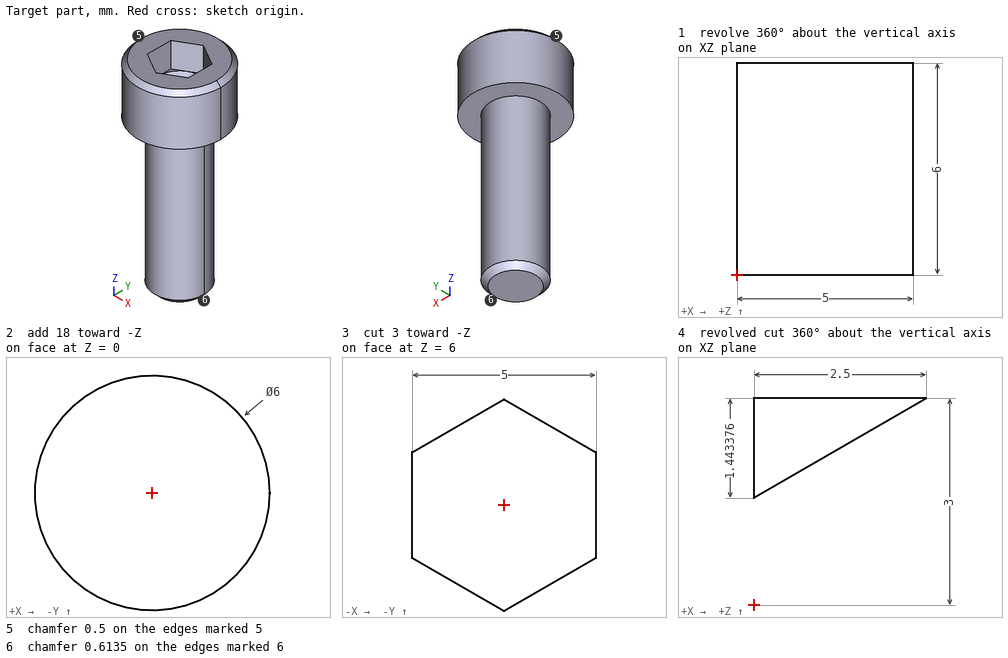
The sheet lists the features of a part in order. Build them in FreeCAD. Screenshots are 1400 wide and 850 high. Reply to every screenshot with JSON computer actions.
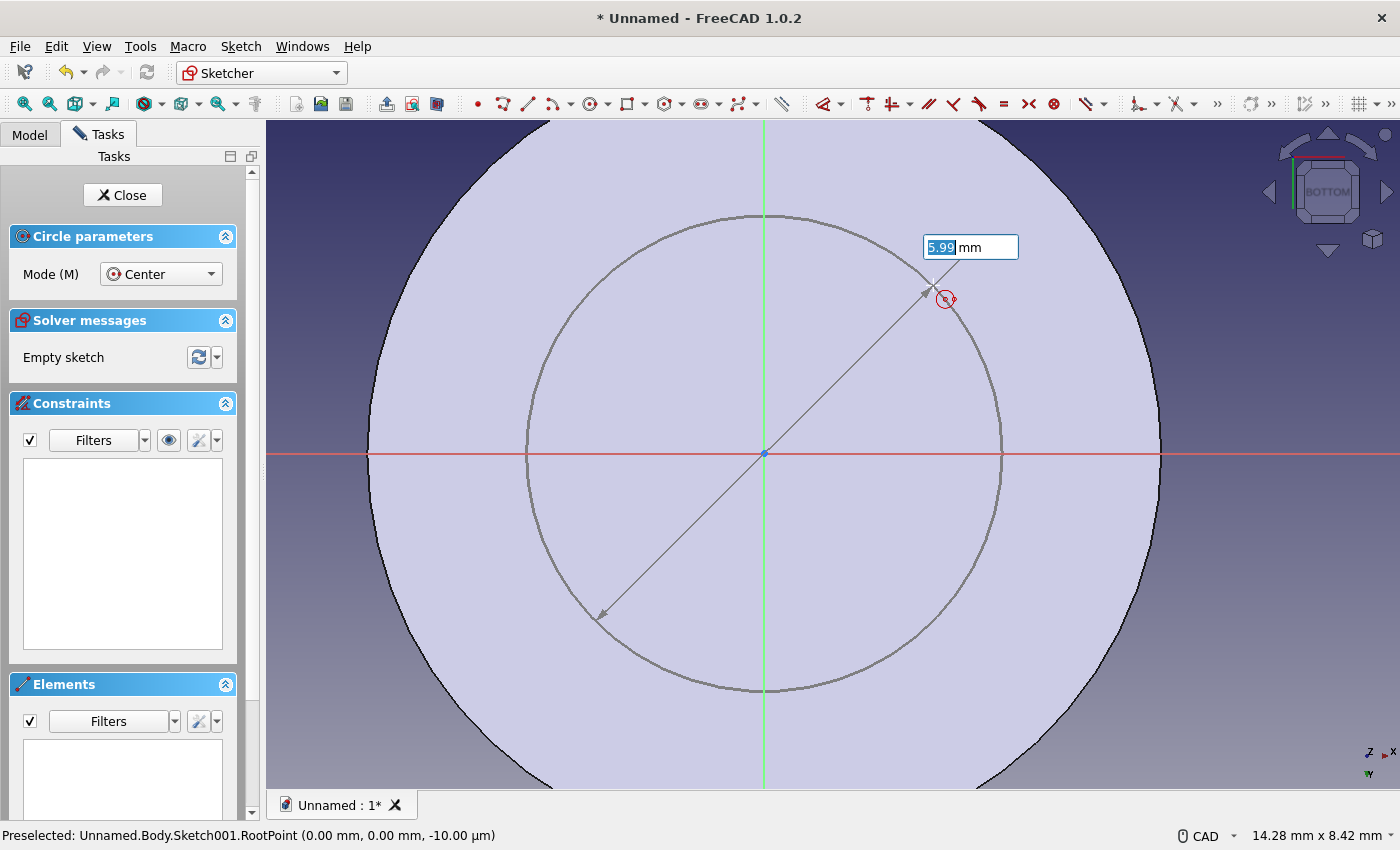
{"action": "type", "text": "6"}
{"action": "key", "text": "Return"}
{"action": "key", "text": "Escape"}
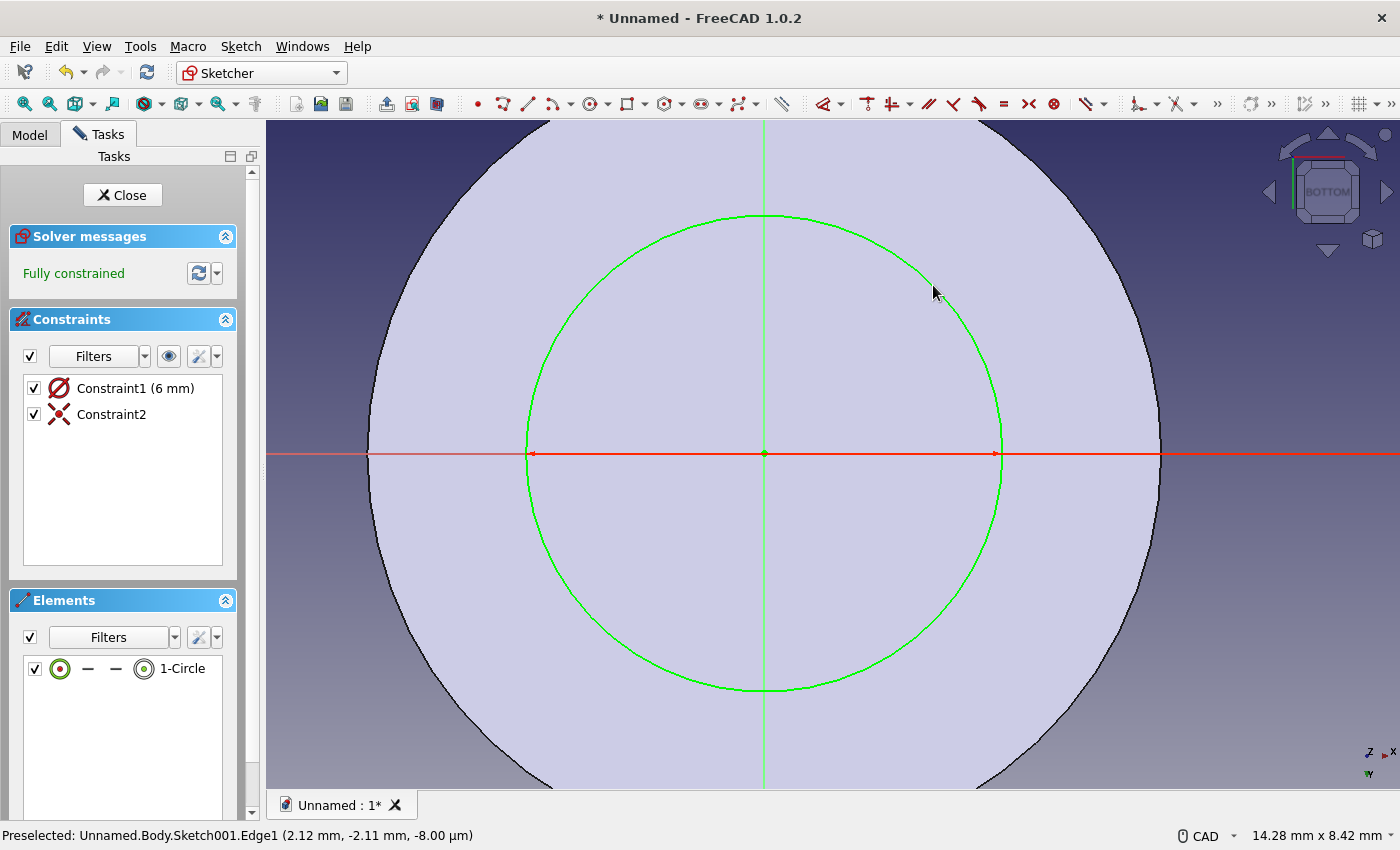
{"action": "left_click", "coordinate": [123, 195]}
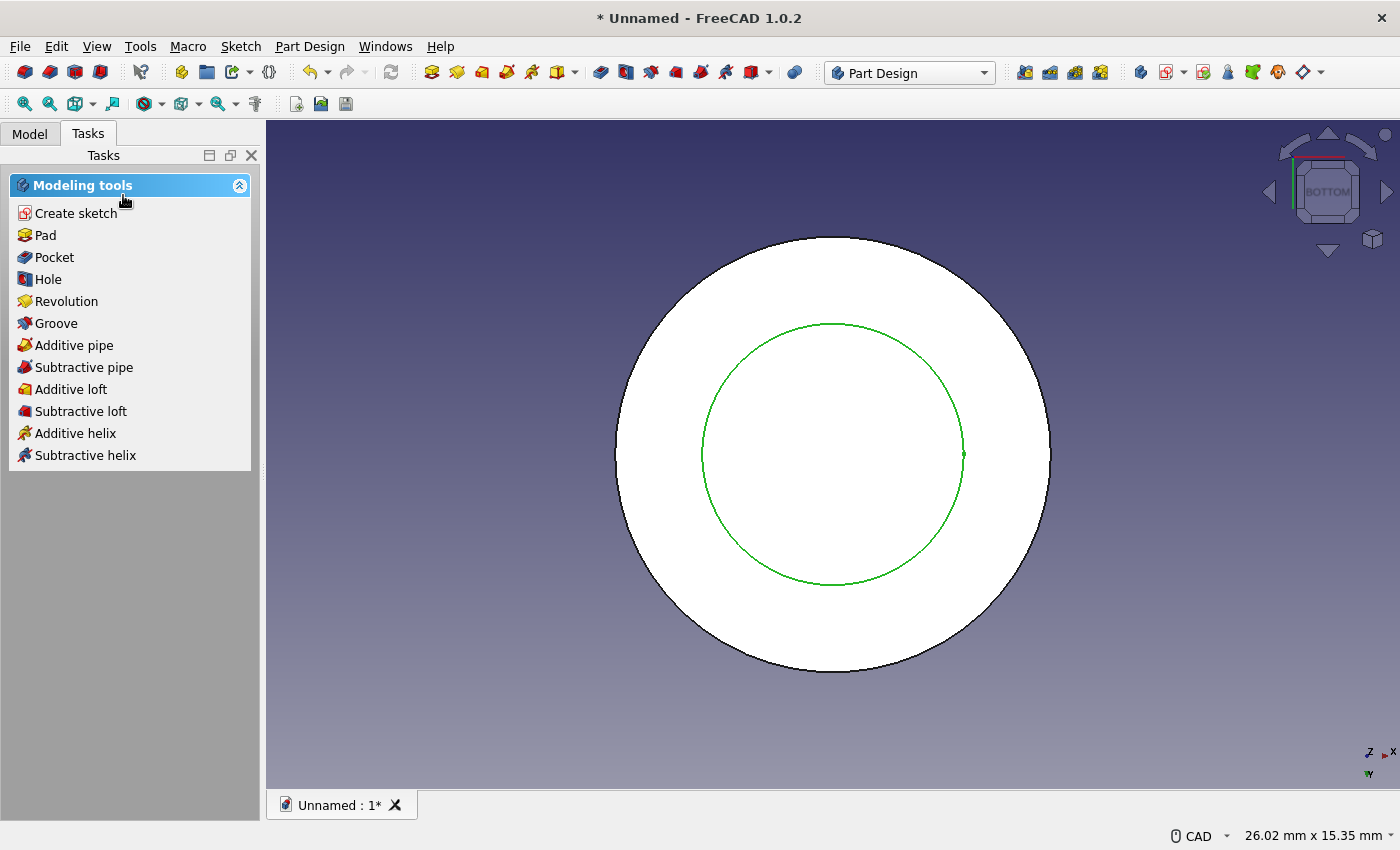
{"action": "left_click", "coordinate": [432, 72]}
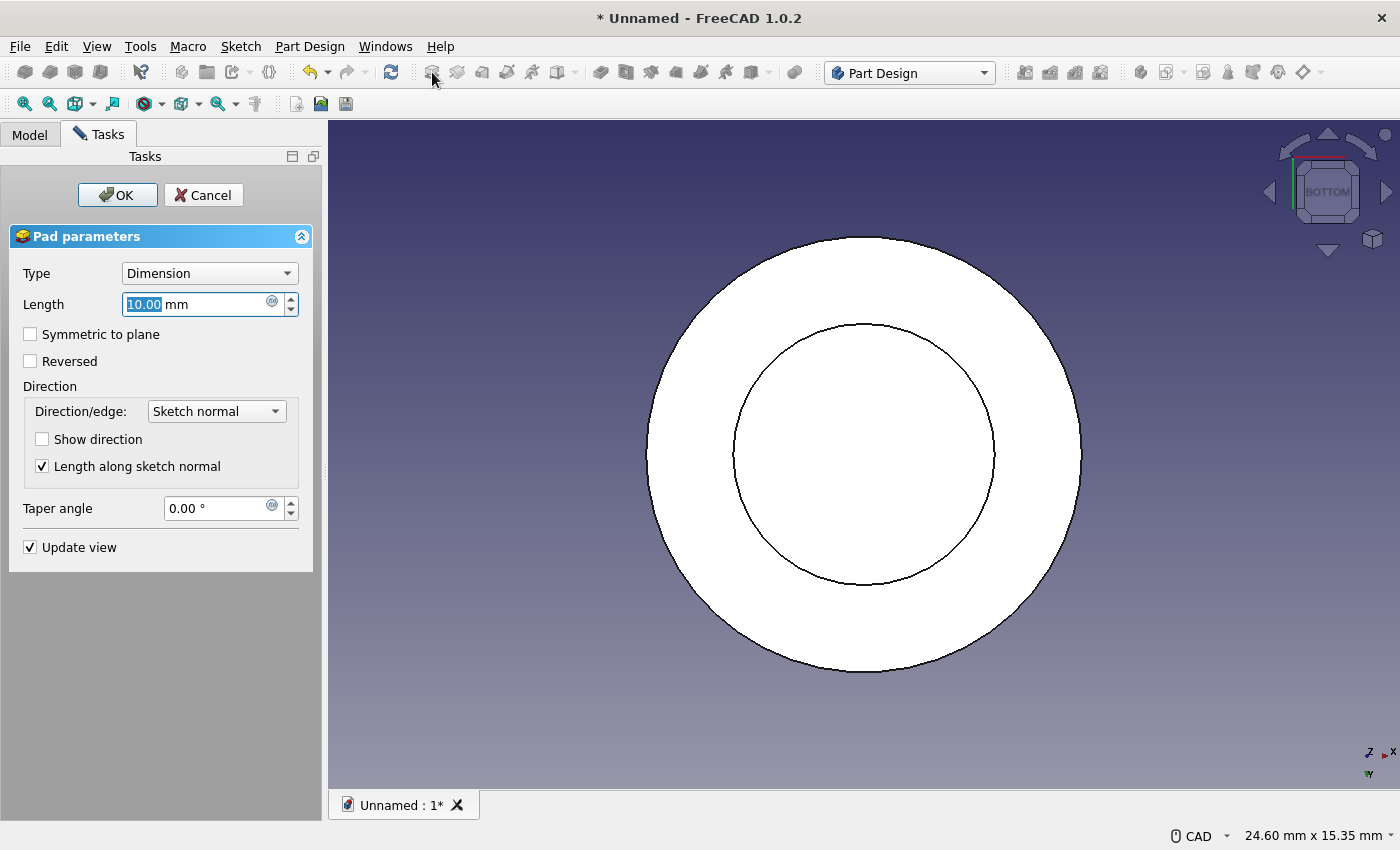
{"action": "type", "text": "18"}
{"action": "key", "text": "Tab"}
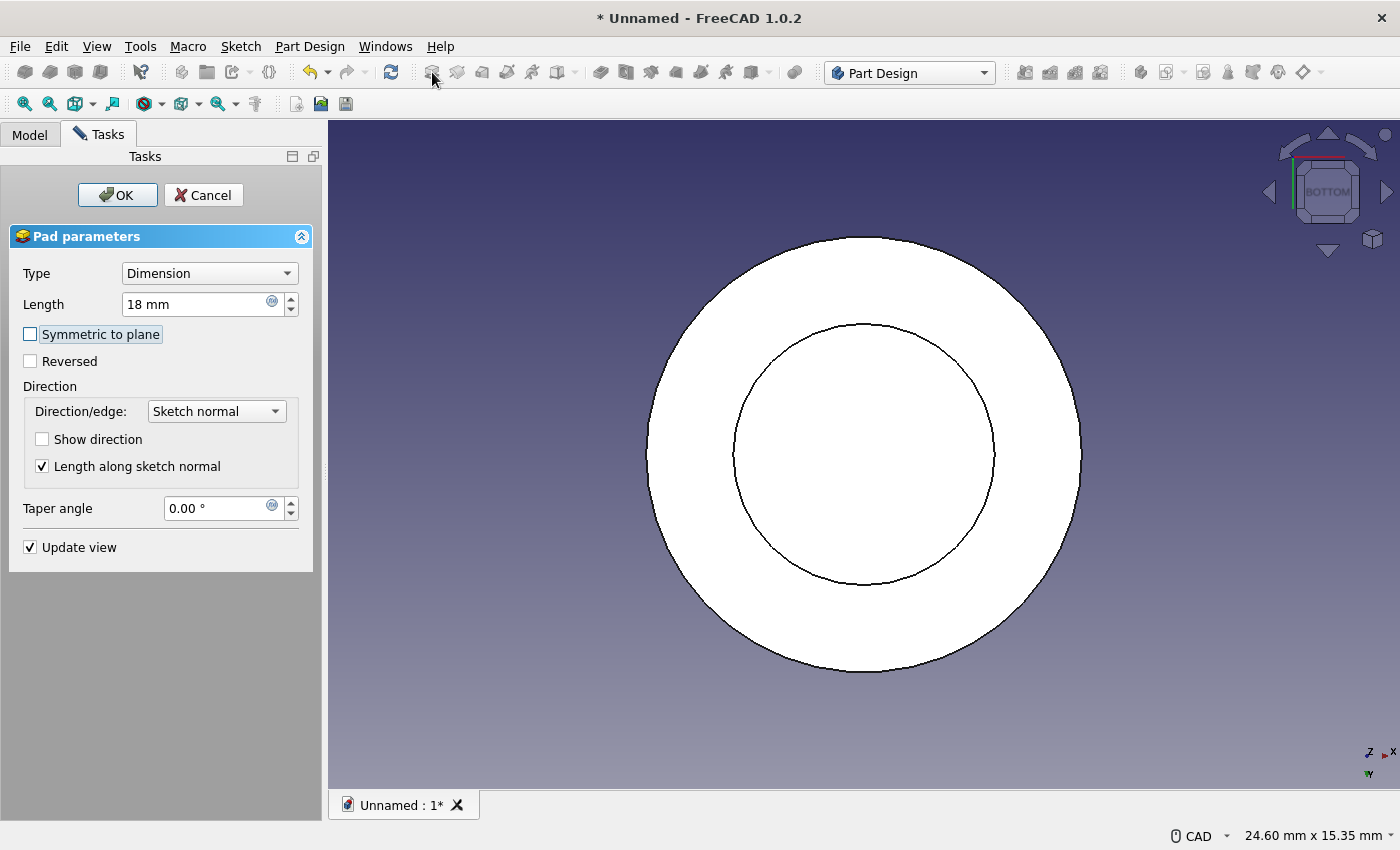
{"action": "left_click", "coordinate": [118, 195]}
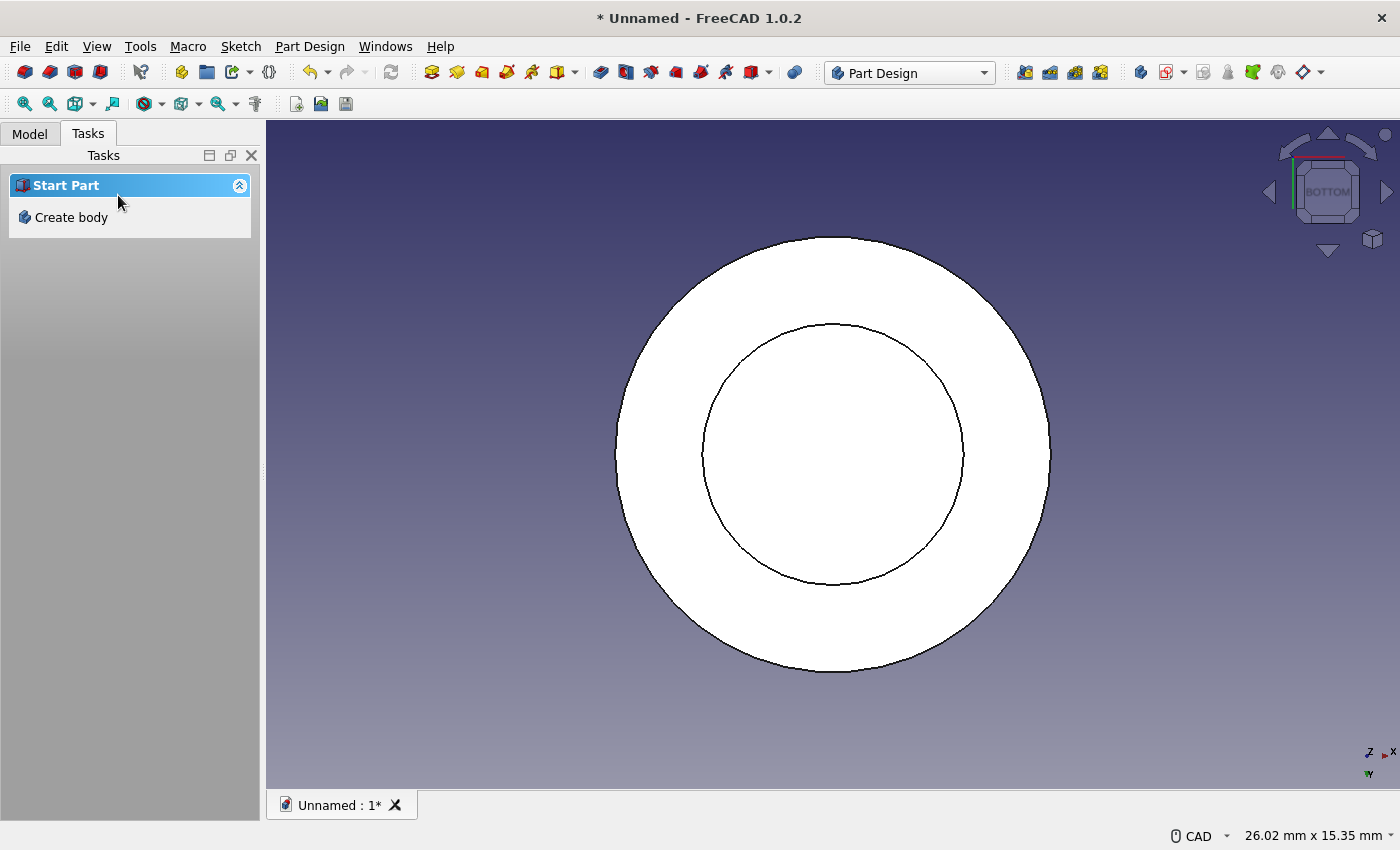
{"action": "key", "text": "0"}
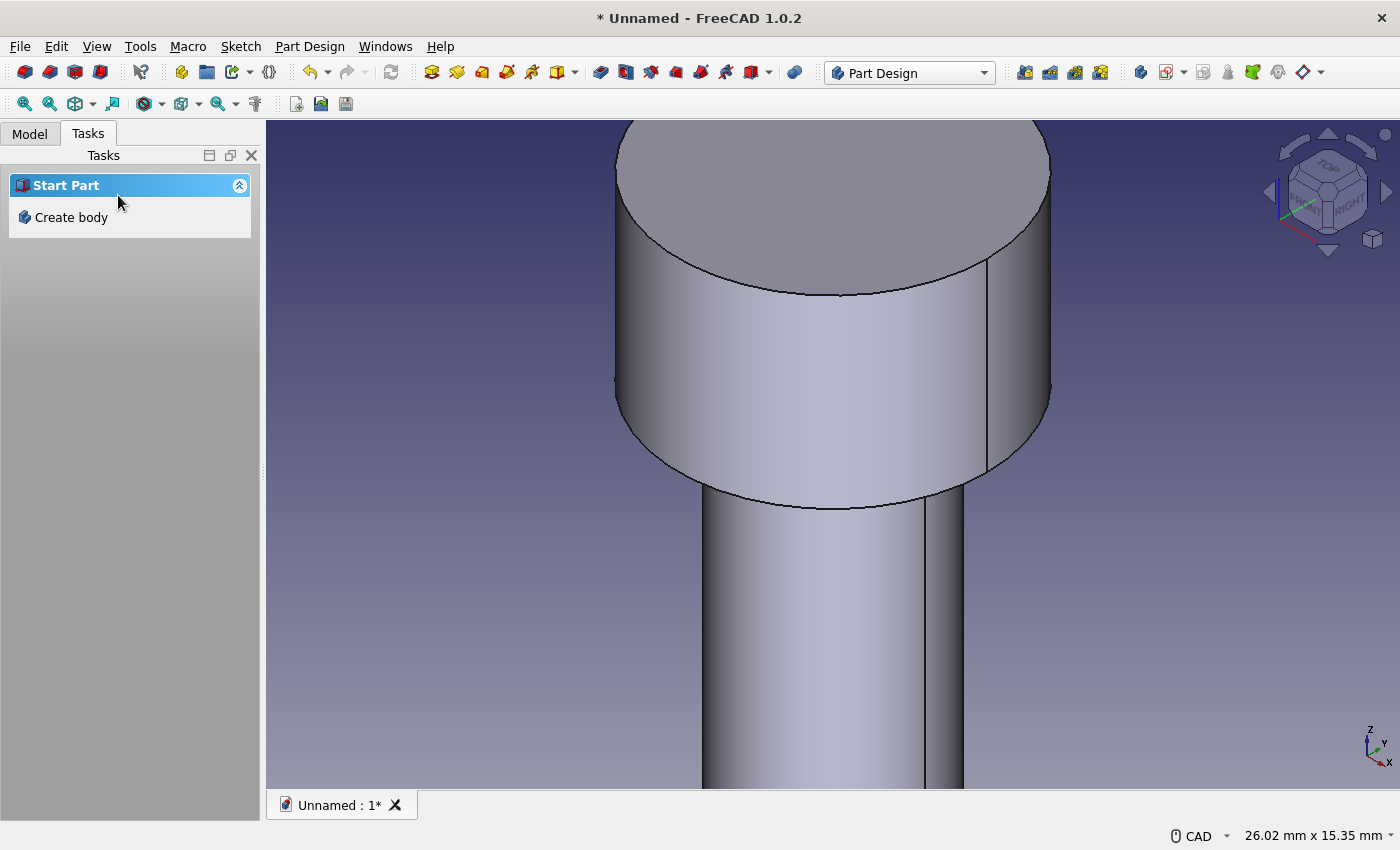
{"action": "left_click", "coordinate": [25, 104]}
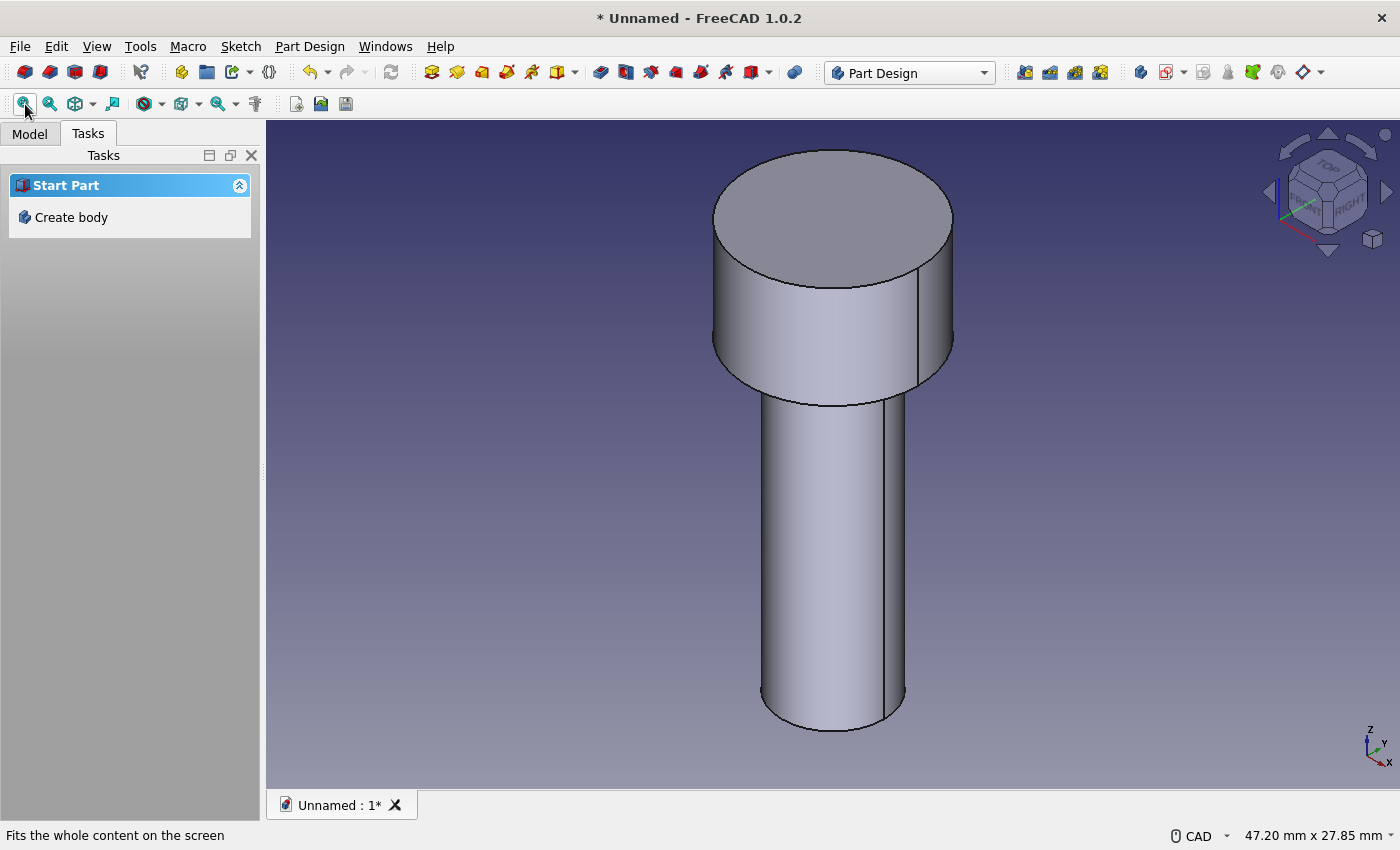
{"action": "left_click", "coordinate": [833, 218]}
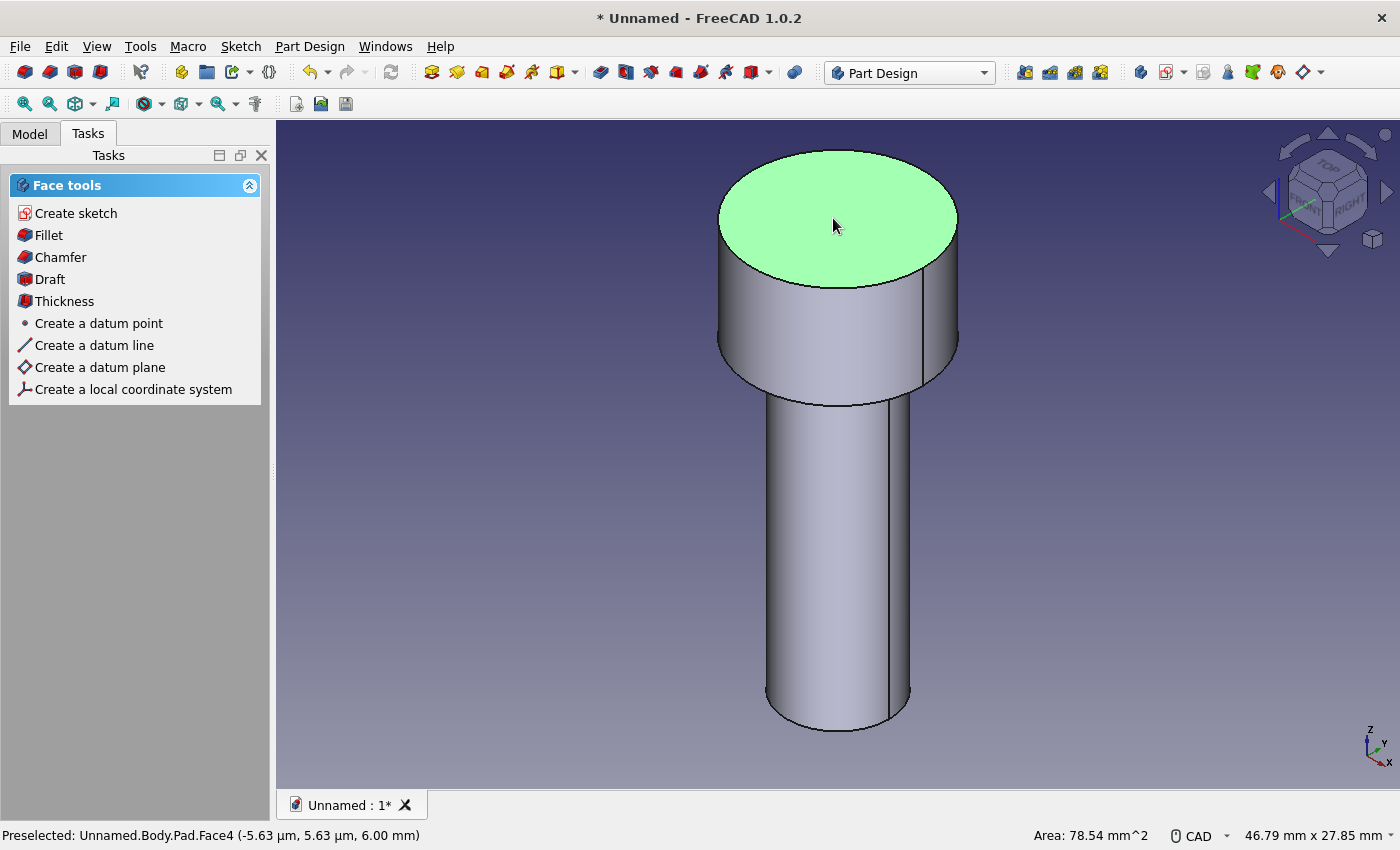
{"action": "left_click", "coordinate": [1166, 72]}